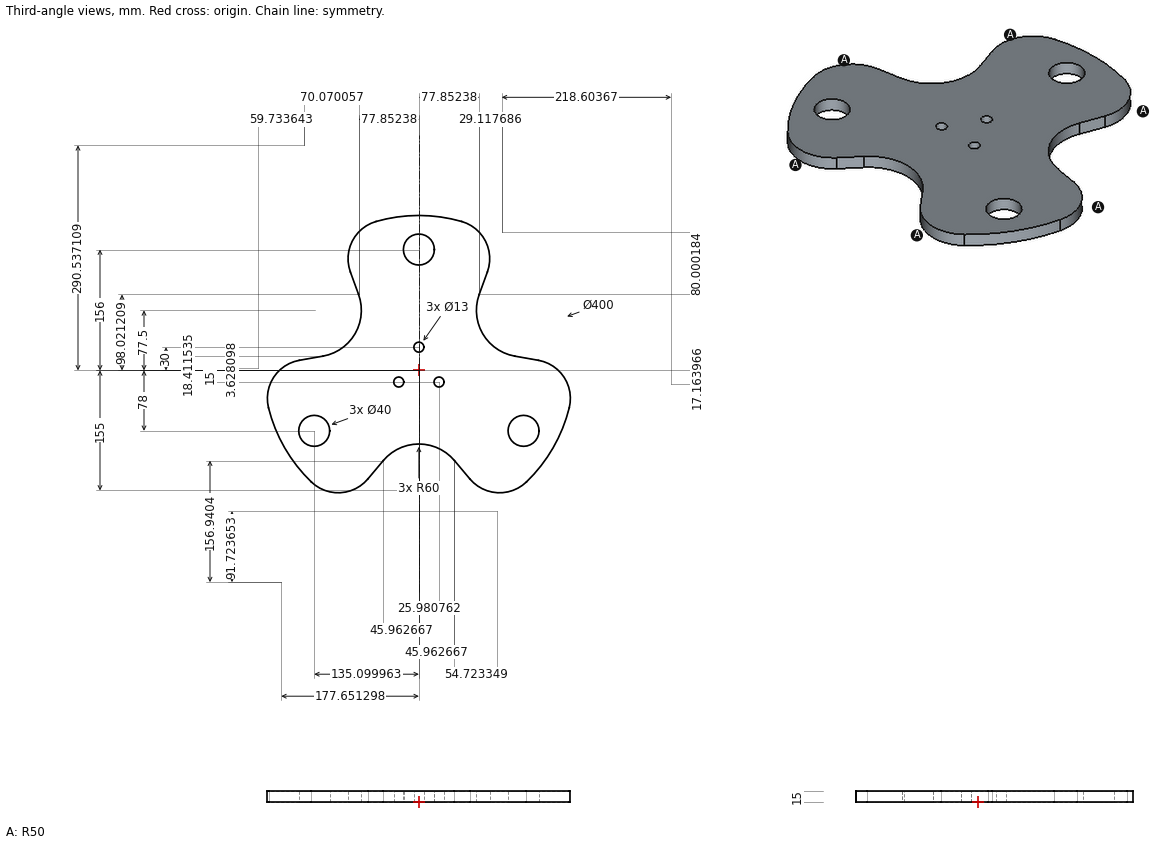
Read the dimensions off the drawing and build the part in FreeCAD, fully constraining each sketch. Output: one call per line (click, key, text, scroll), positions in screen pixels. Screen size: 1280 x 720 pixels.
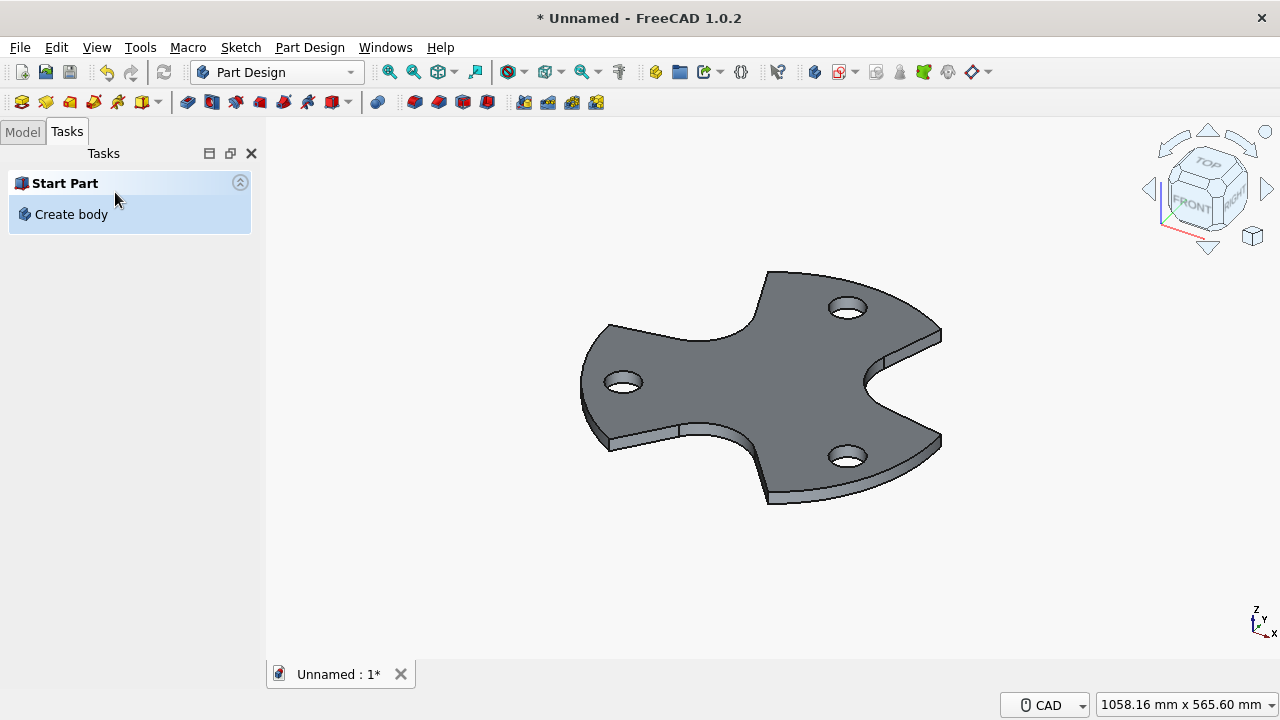
click(609, 445)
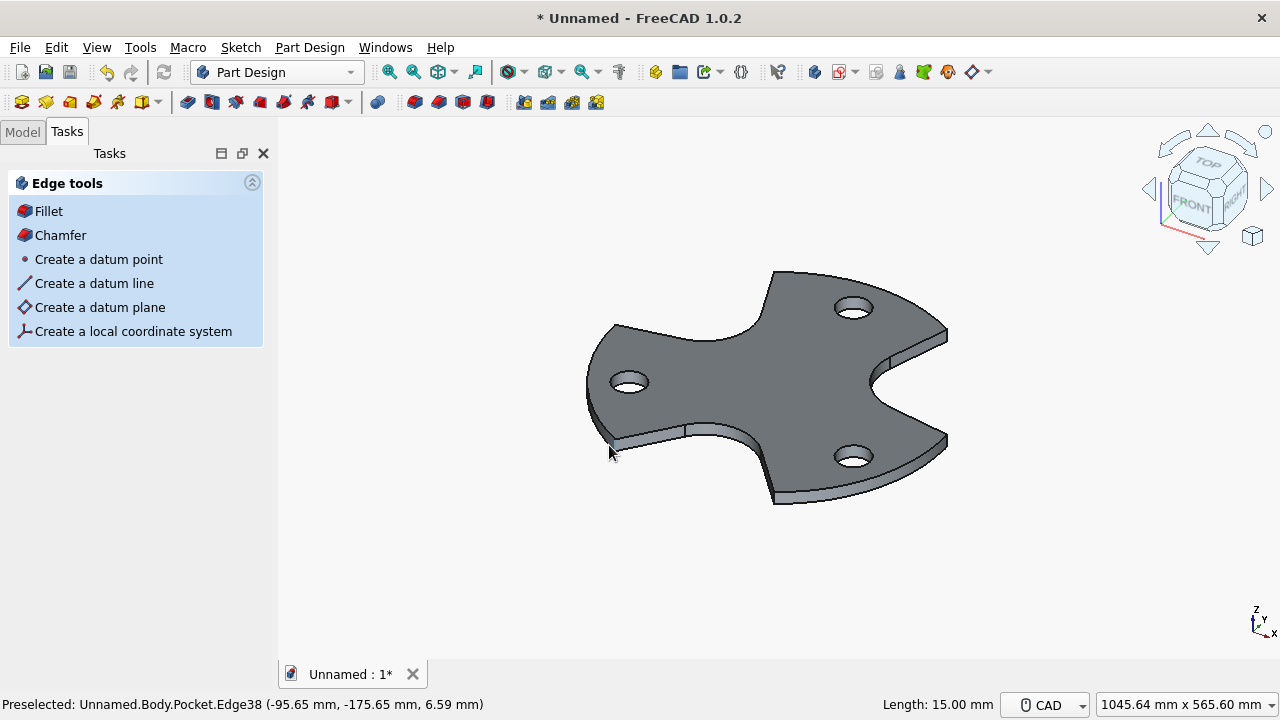
click(774, 497, ctrl)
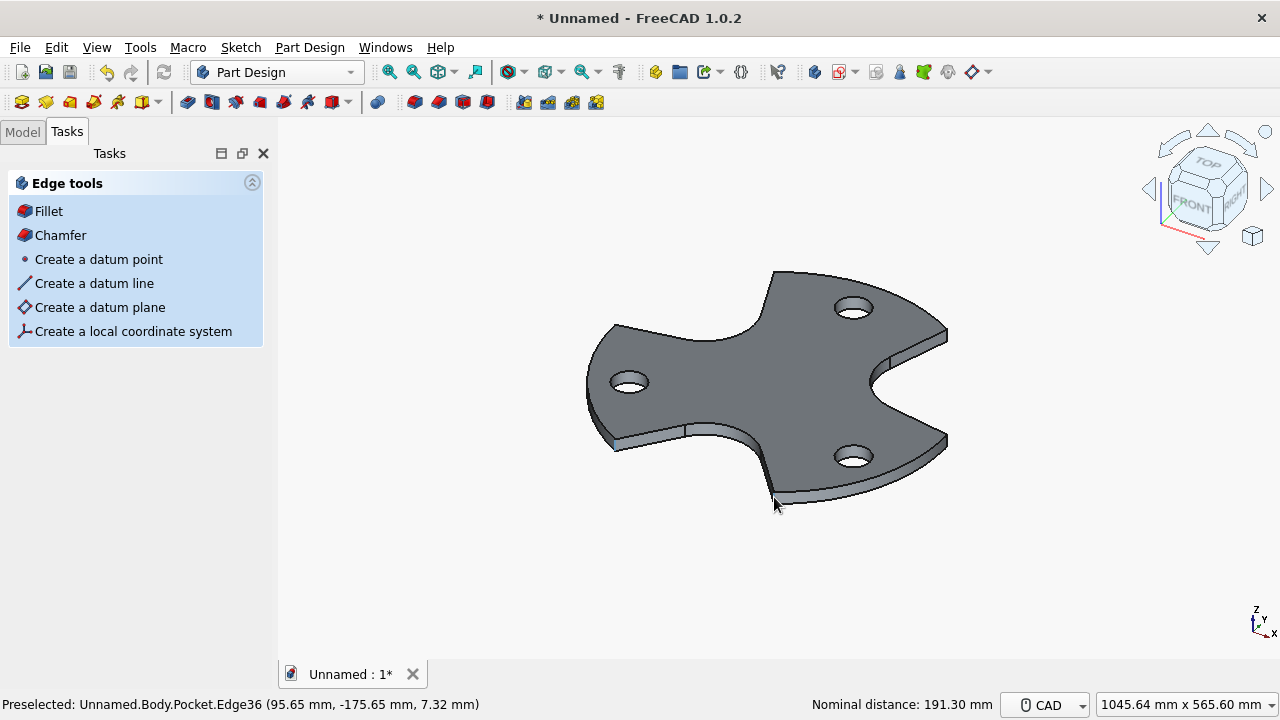
scroll(947, 440, up, 6)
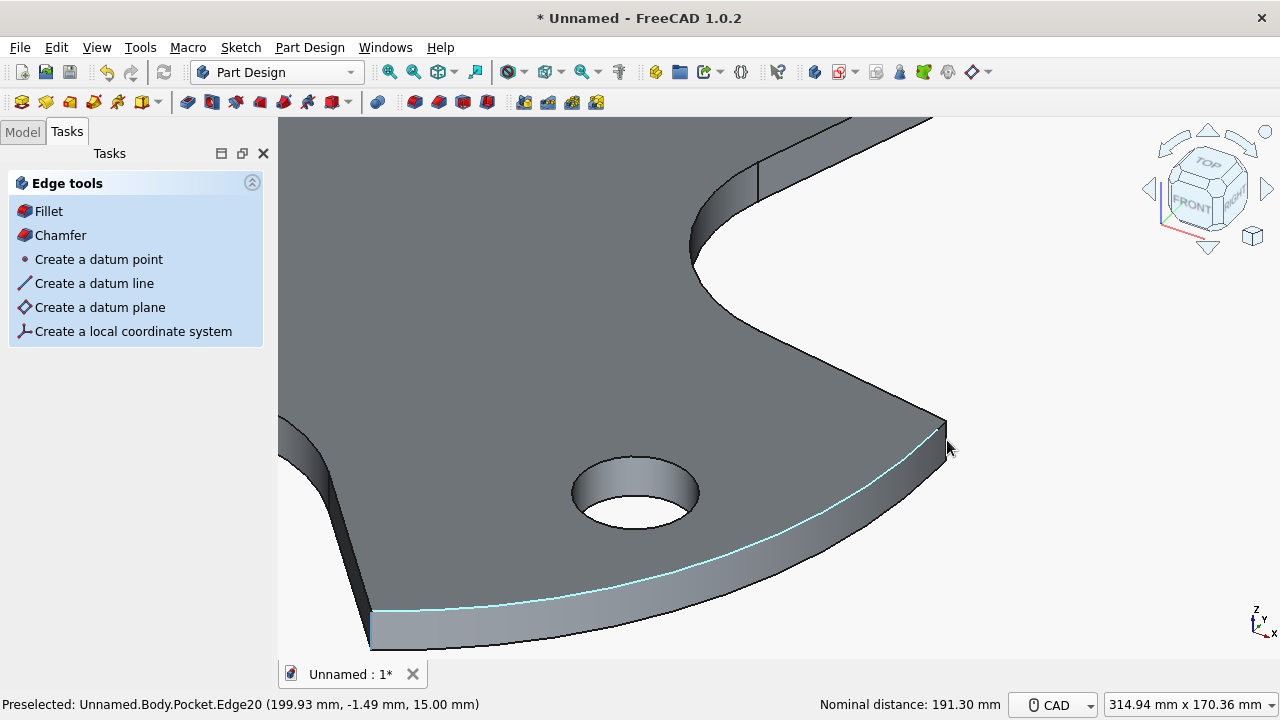
click(390, 72)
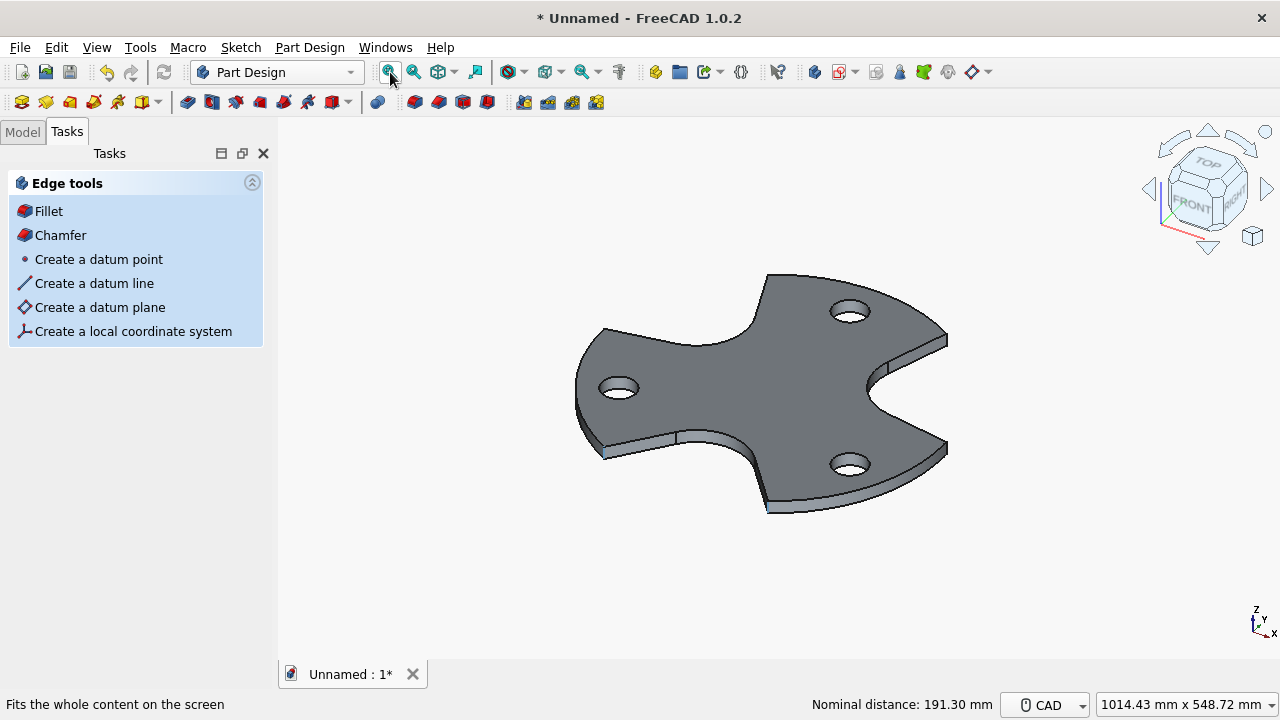
key(0)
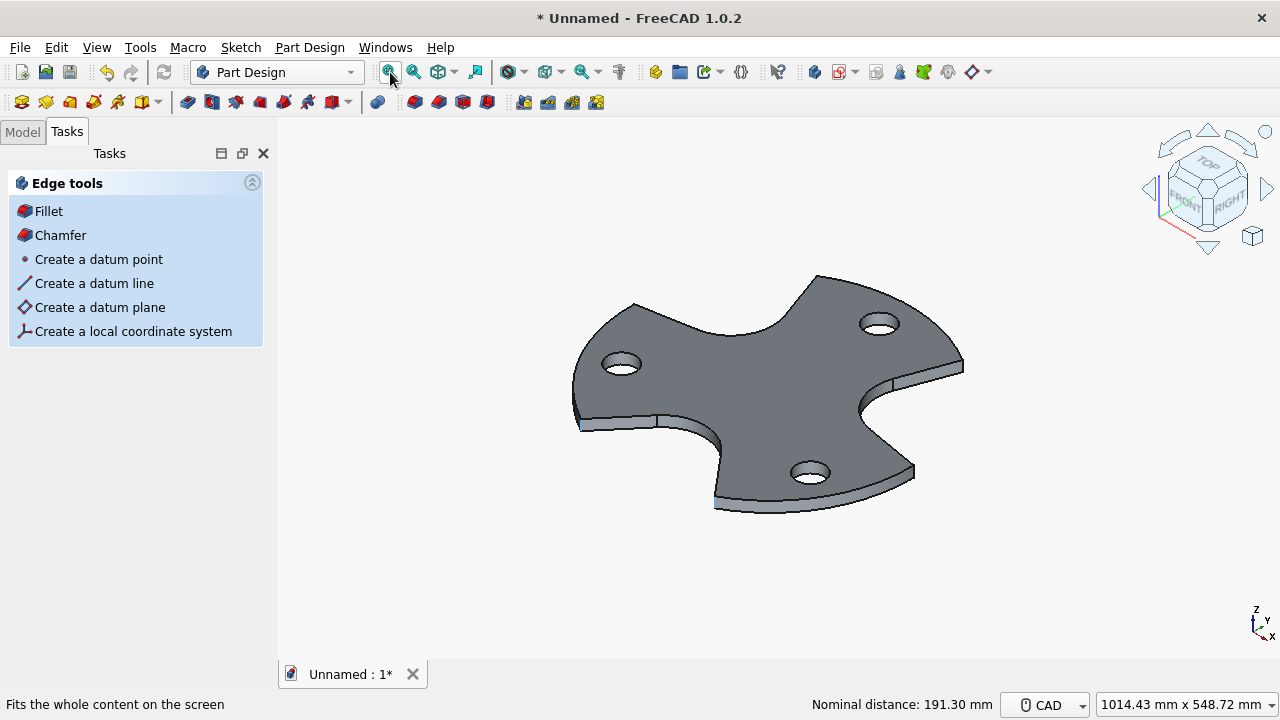
scroll(914, 470, up, 5)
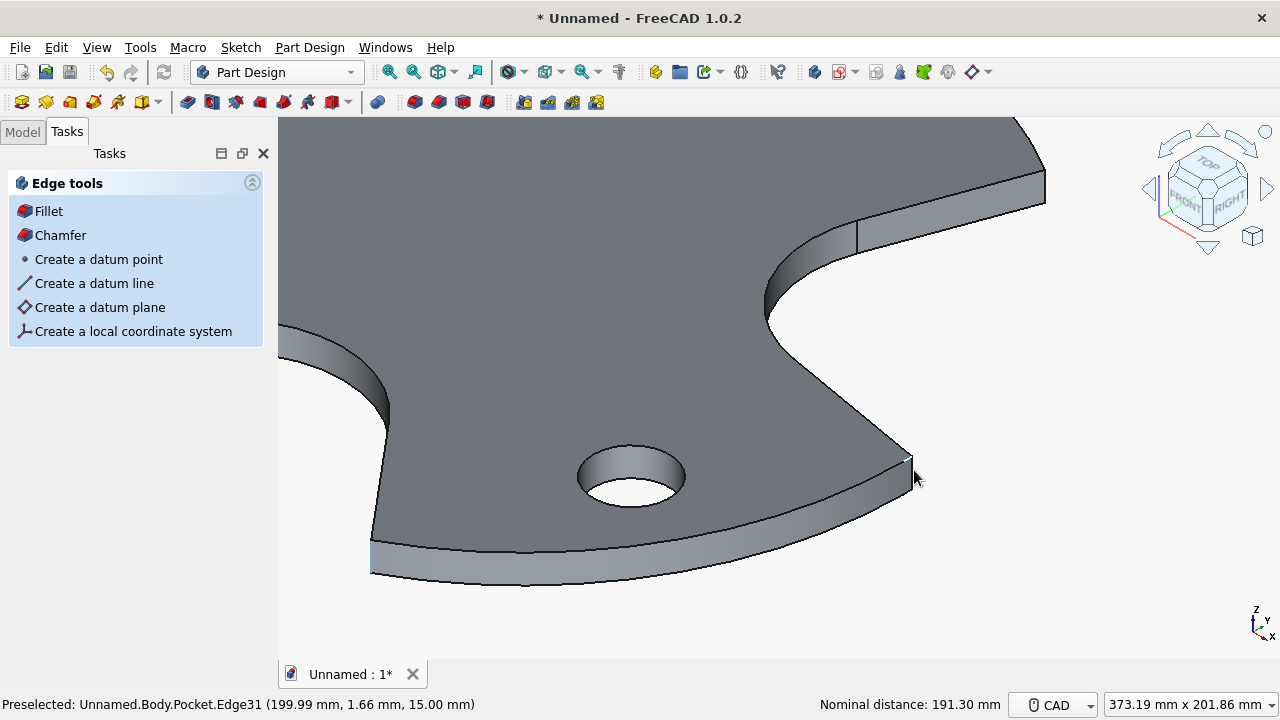
click(390, 72)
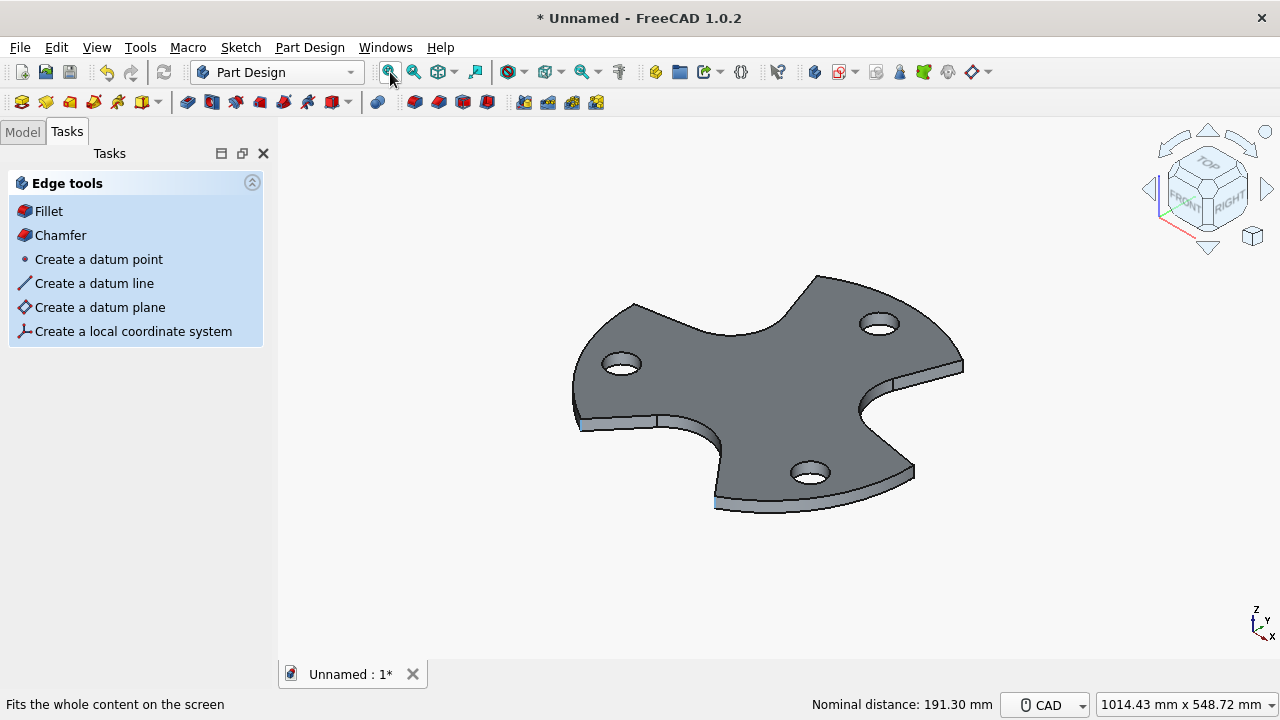
key(2)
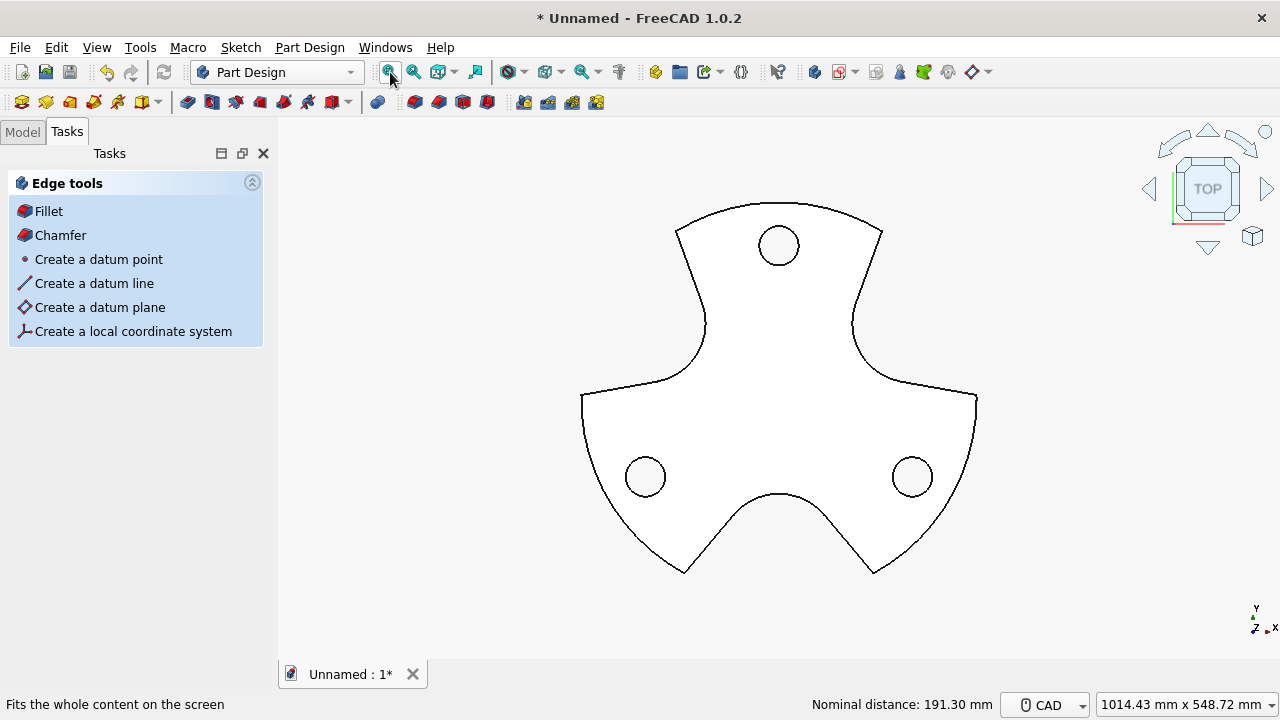
scroll(976, 394, up, 5)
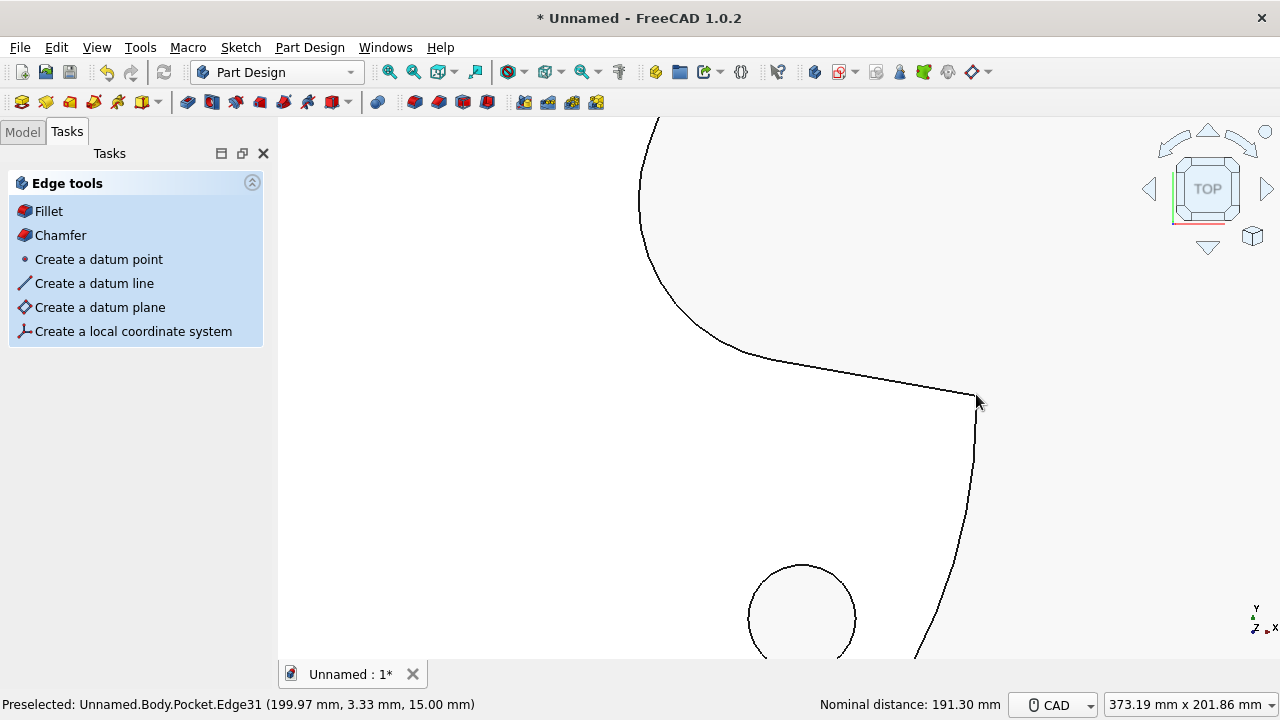
click(390, 72)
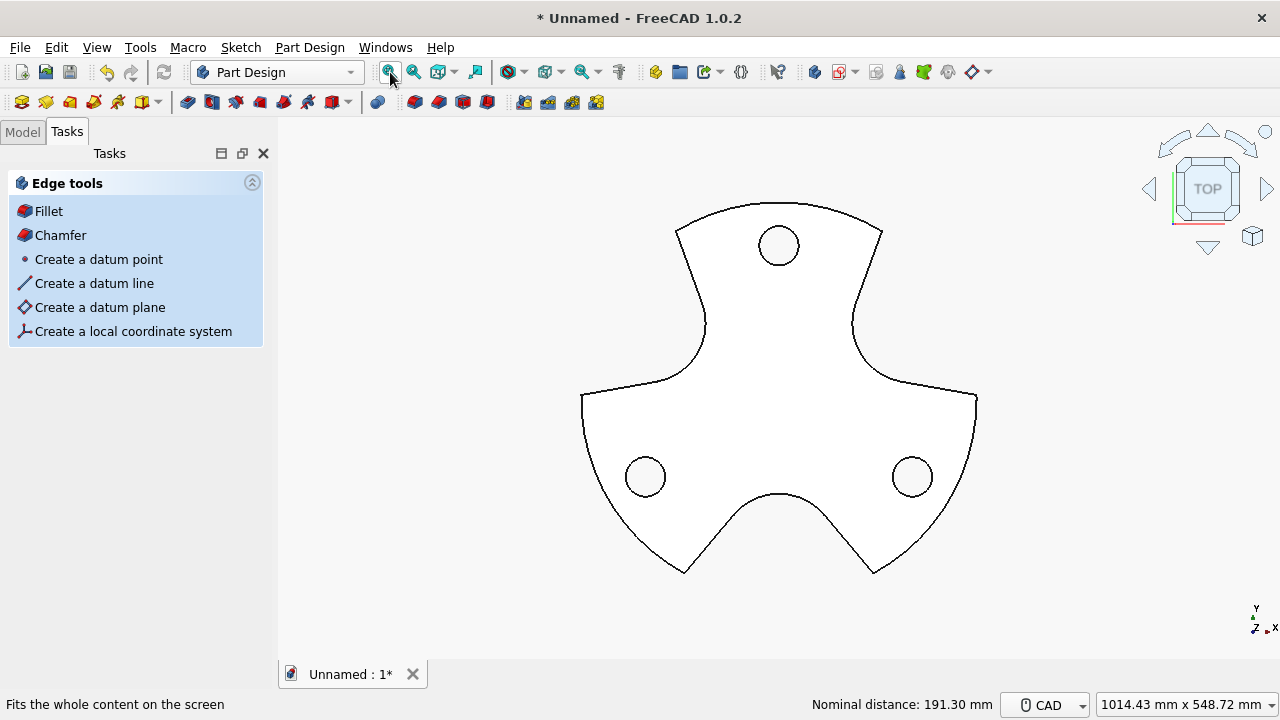
key(1)